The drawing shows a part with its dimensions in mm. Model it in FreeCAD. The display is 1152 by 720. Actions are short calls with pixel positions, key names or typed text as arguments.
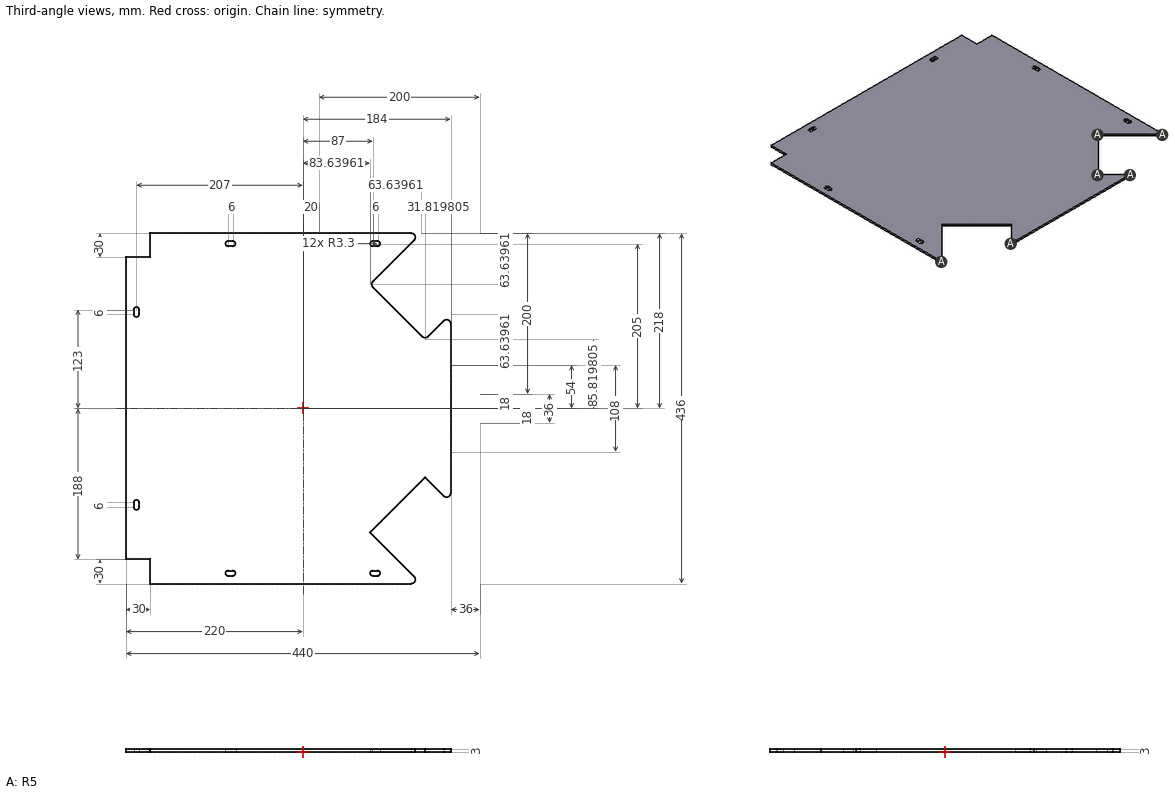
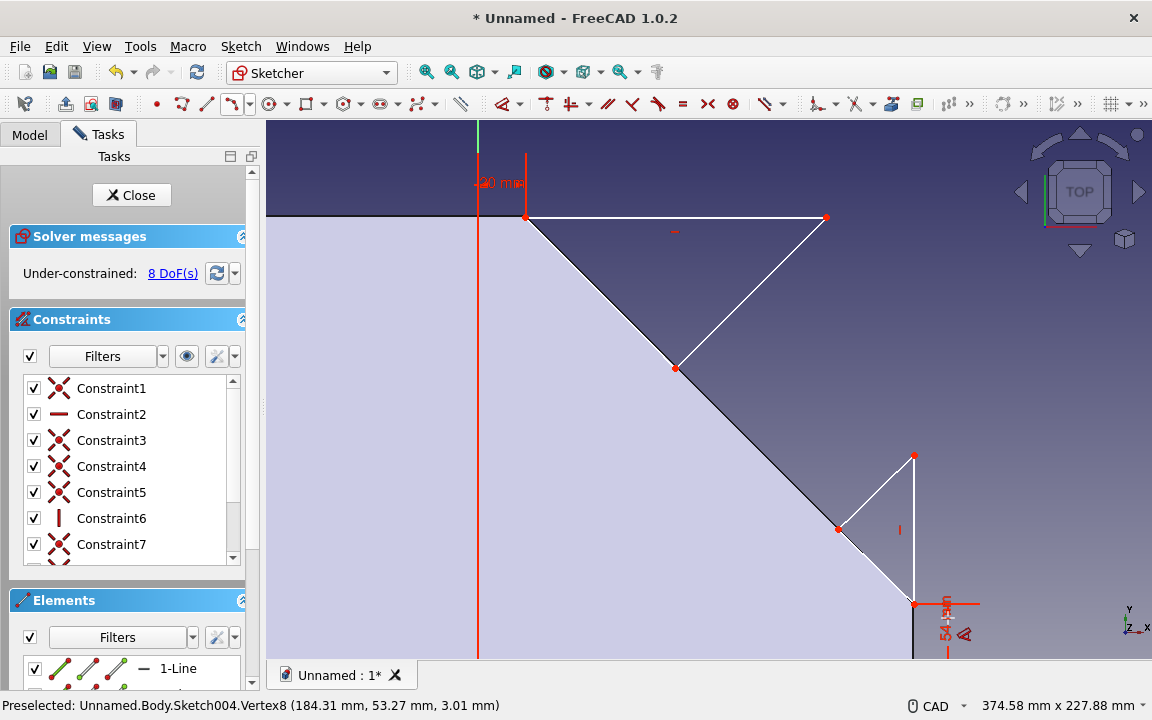
click(826, 218)
click(444, 424)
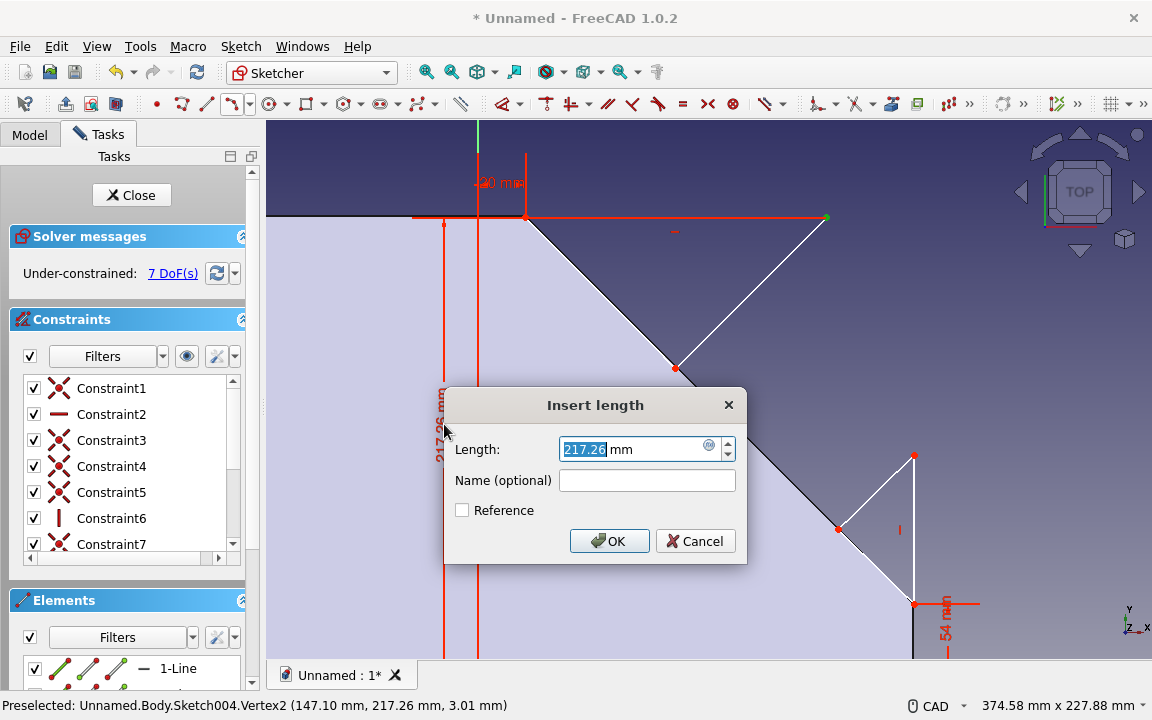
text(218)
key(Return)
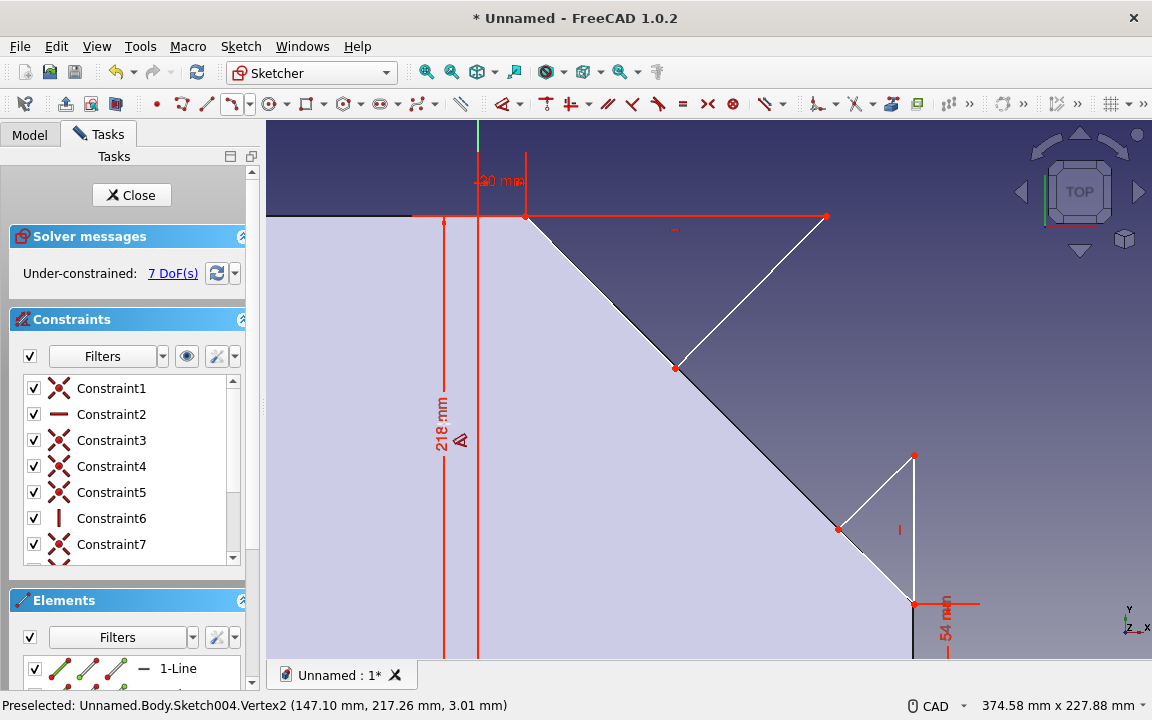
click(914, 604)
click(696, 570)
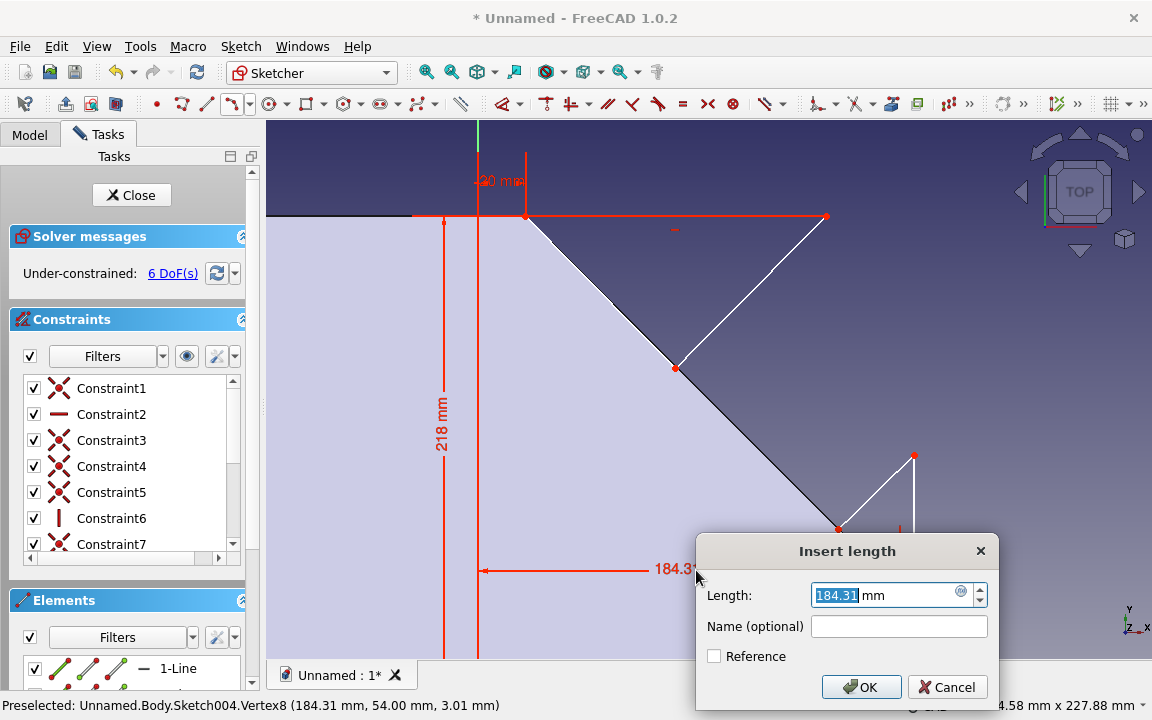
text(184)
key(Return)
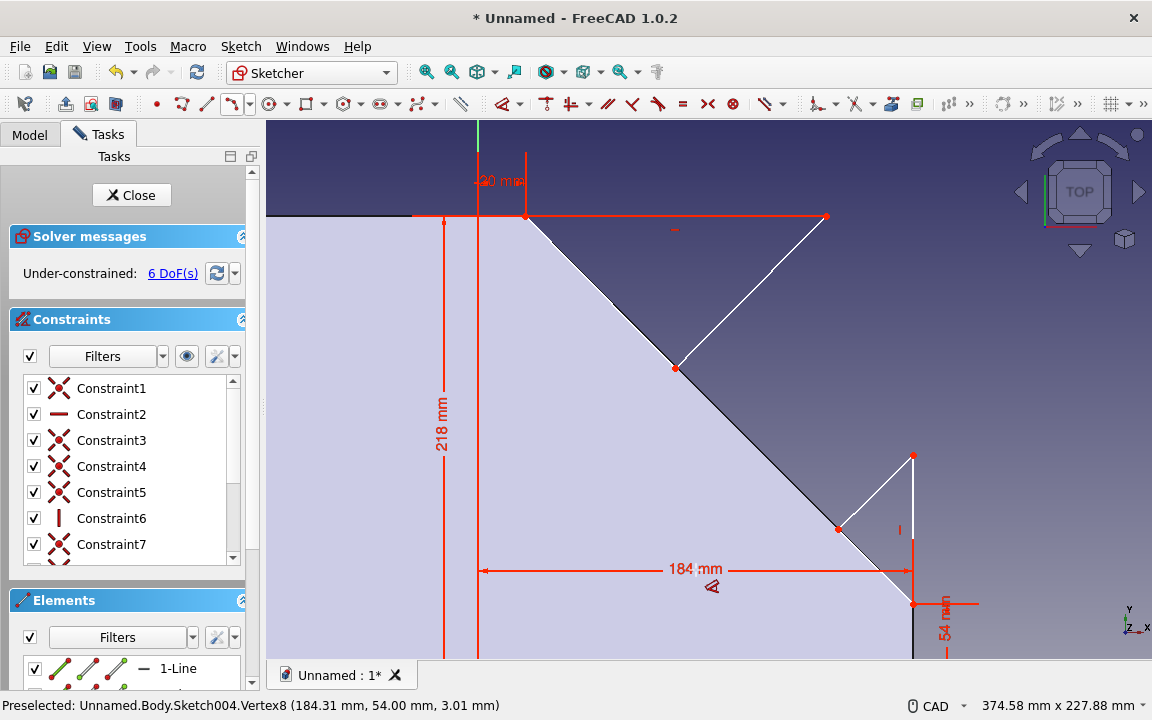
click(913, 559)
click(947, 530)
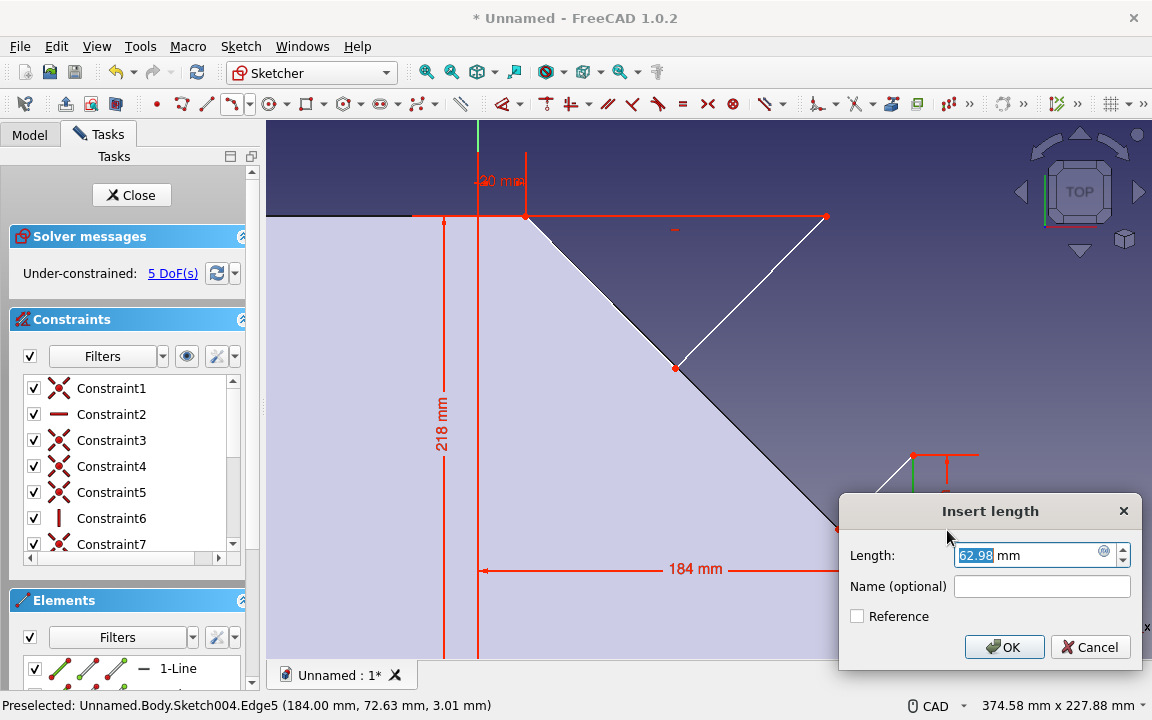
text(63.63961)
key(Return)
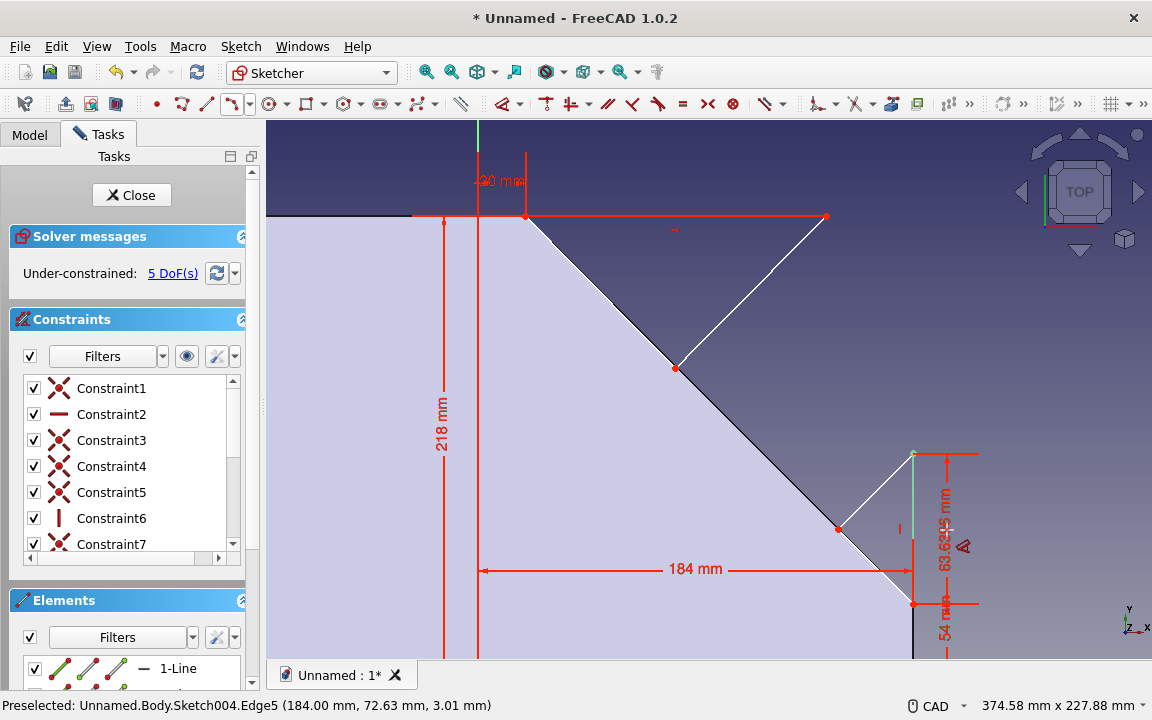
click(676, 369)
click(577, 335)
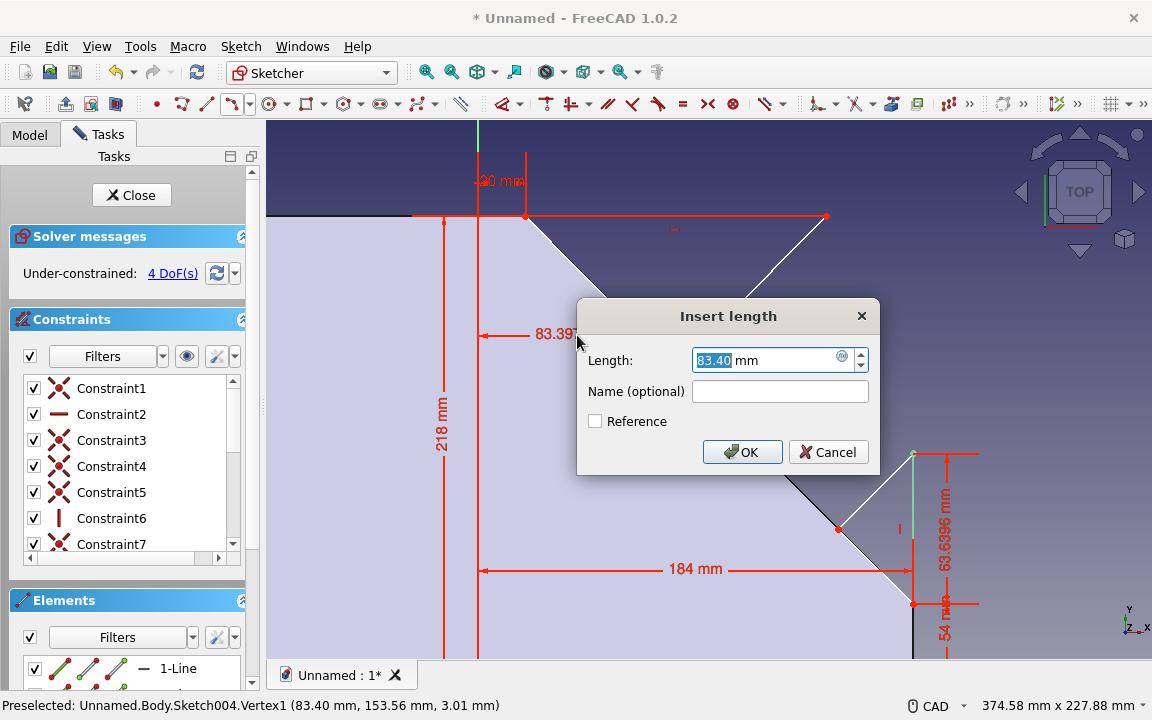
text(83.63961)
key(Return)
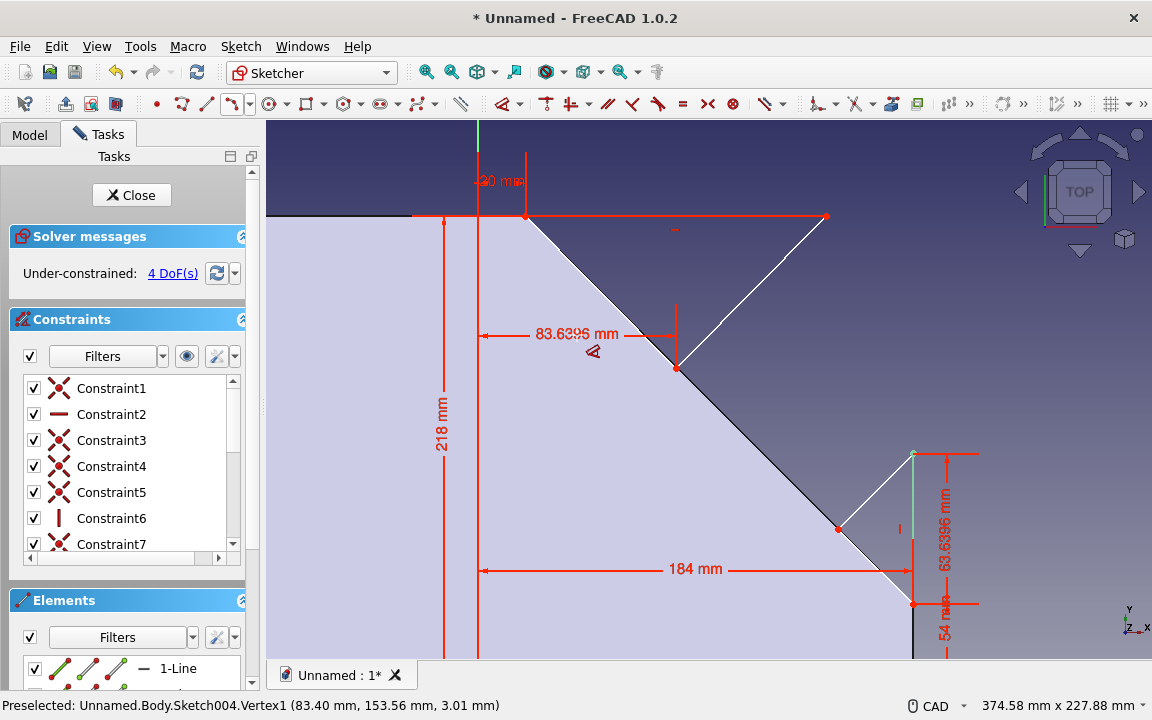
click(721, 323)
click(751, 182)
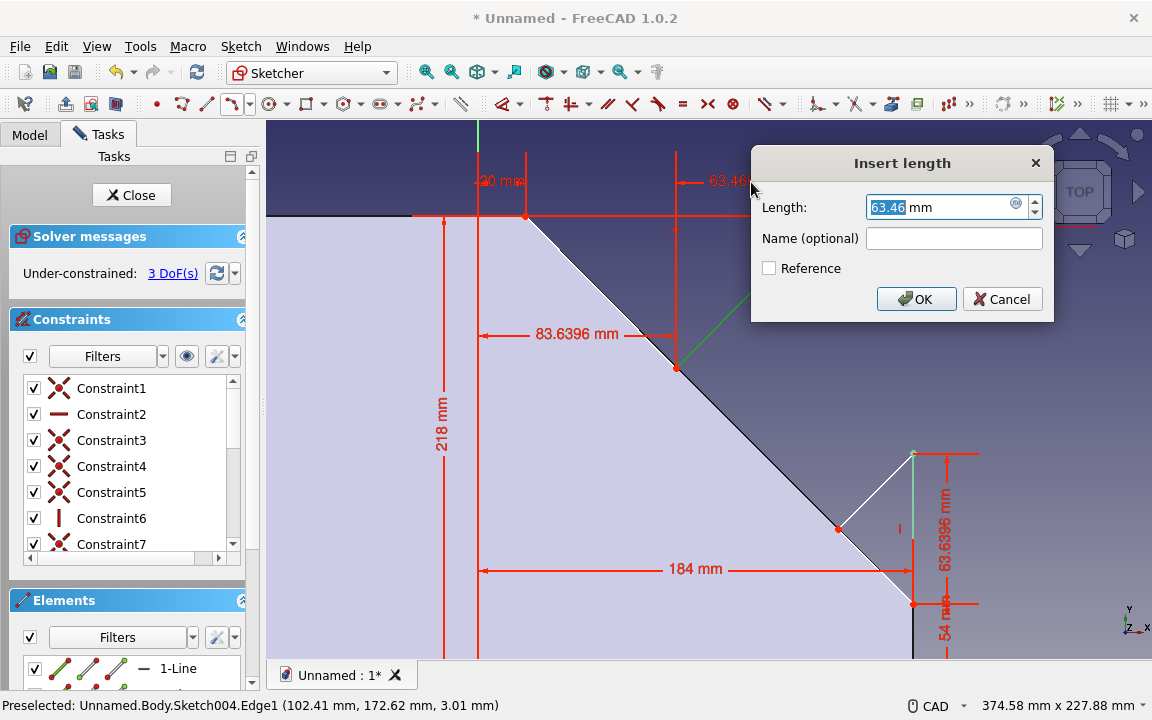
text(63.63961)
key(Return)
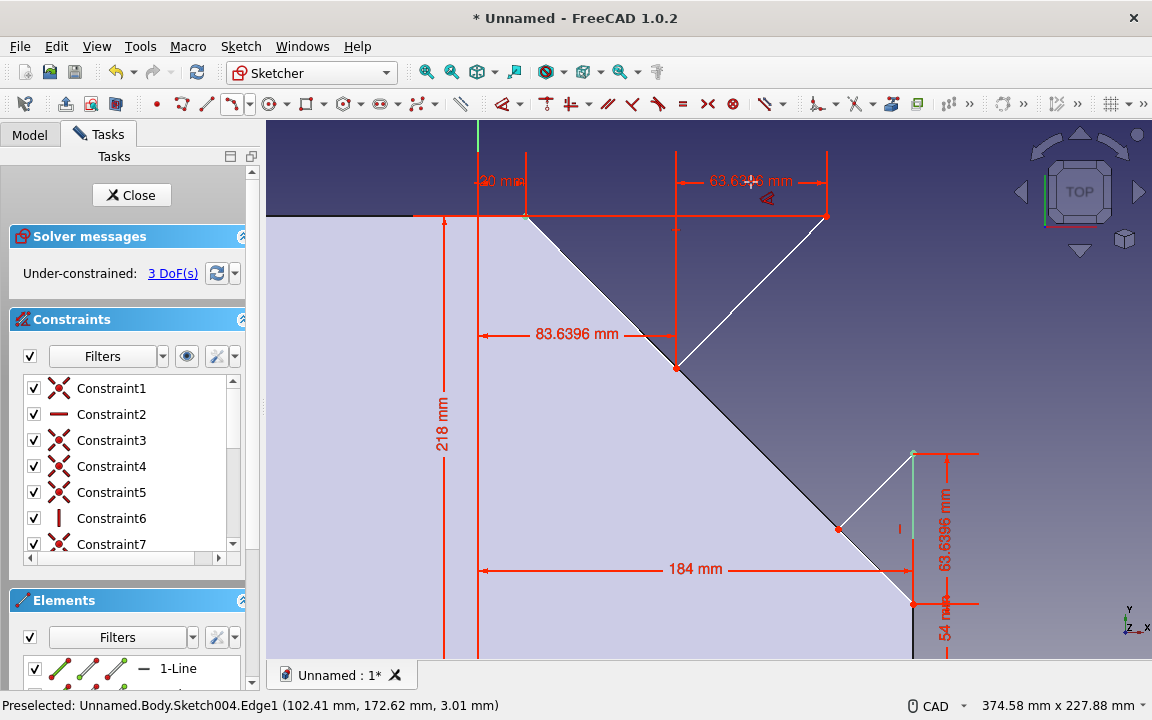
click(721, 323)
click(861, 292)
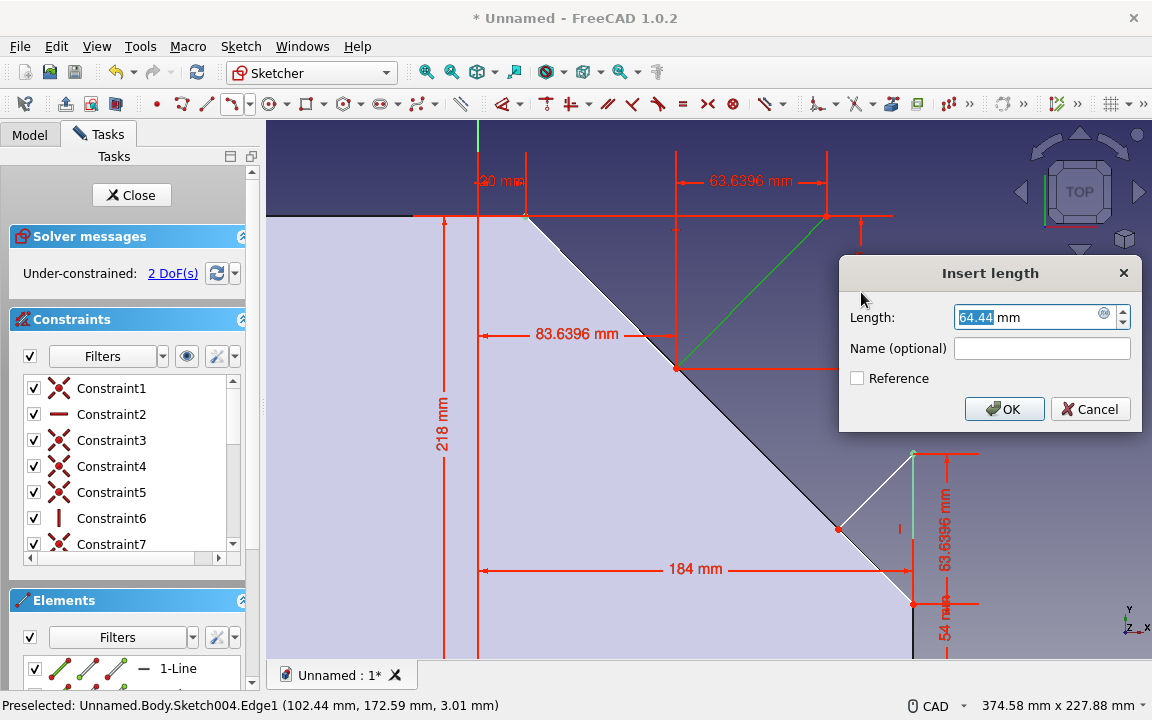
text(63.63961)
key(Return)